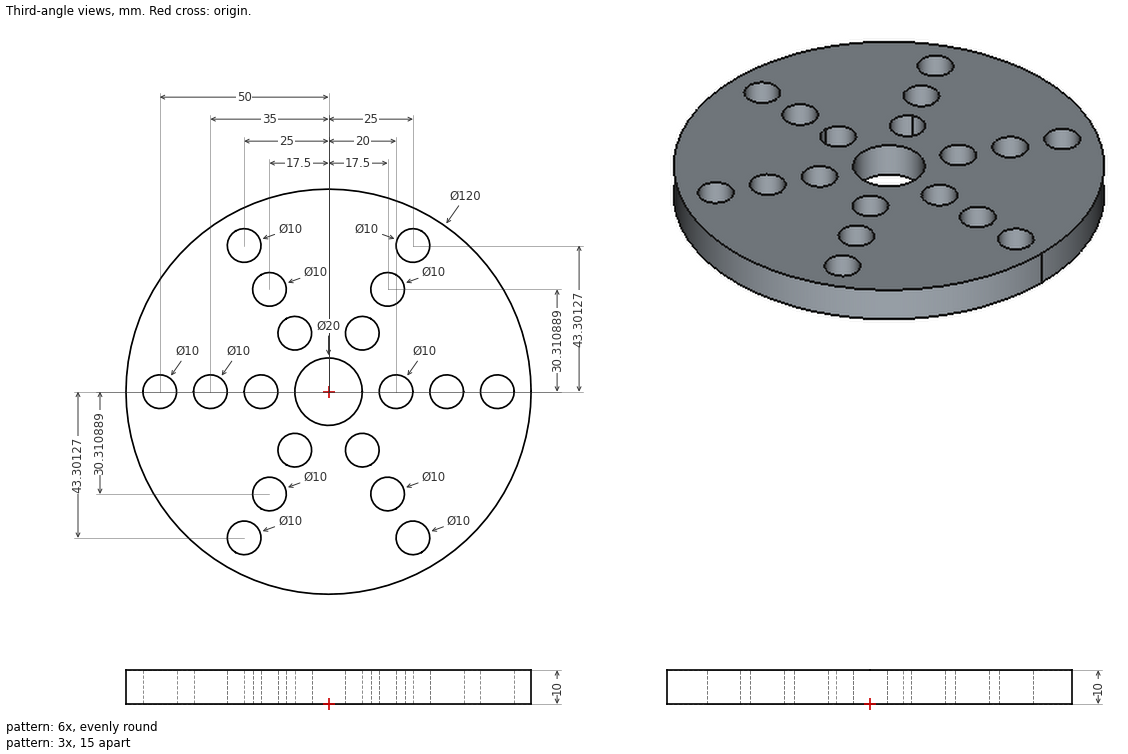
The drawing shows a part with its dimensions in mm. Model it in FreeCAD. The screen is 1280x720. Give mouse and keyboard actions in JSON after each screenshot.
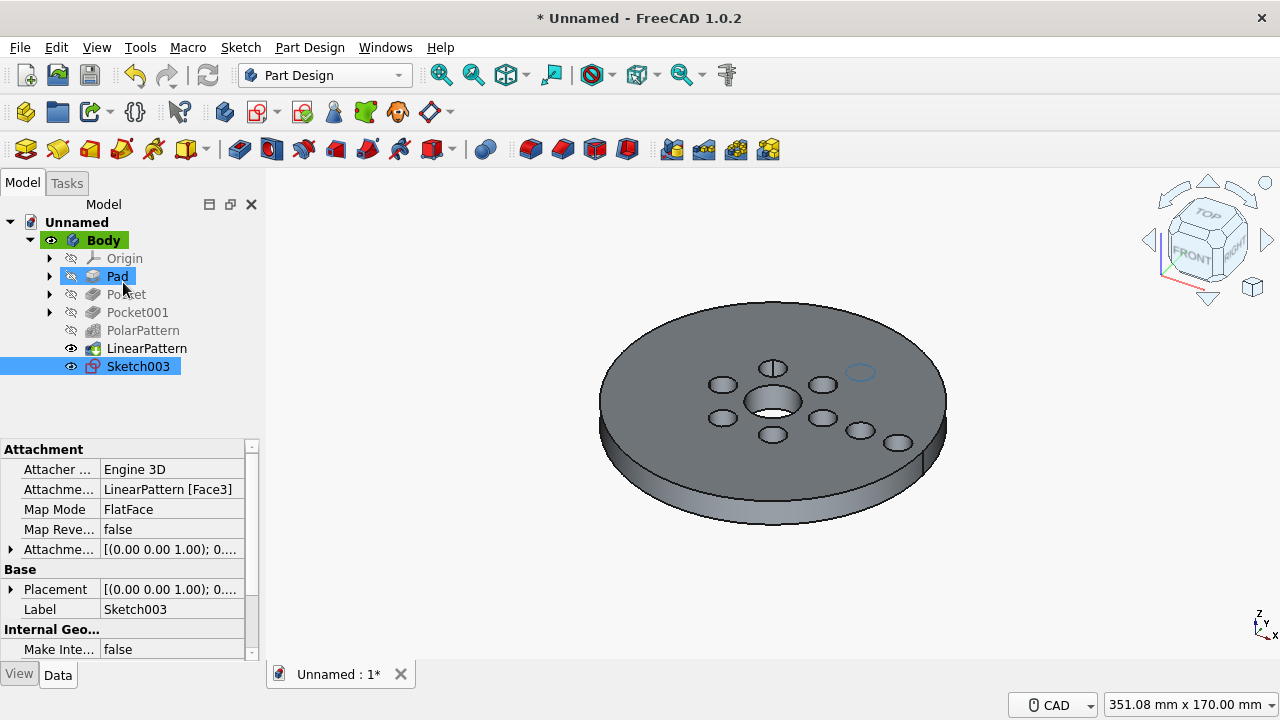
{"action": "left_click", "coordinate": [240, 150]}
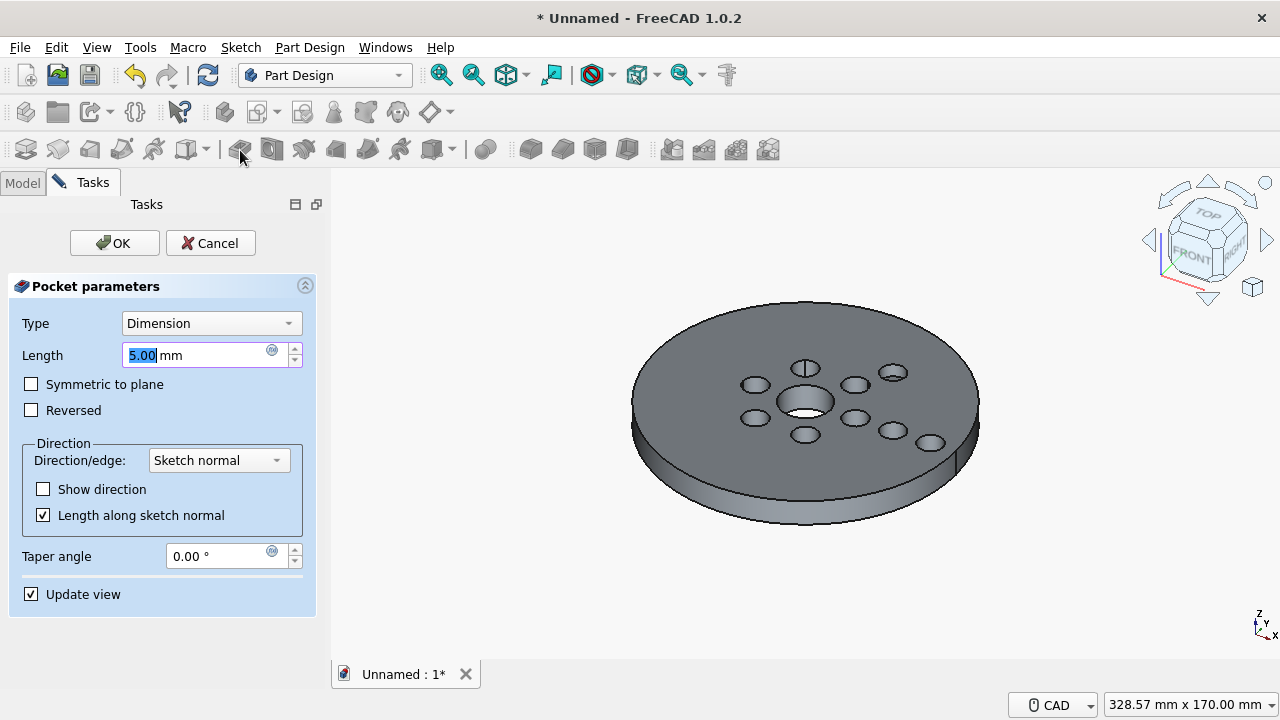
{"action": "type", "text": "10"}
{"action": "key", "text": "Tab"}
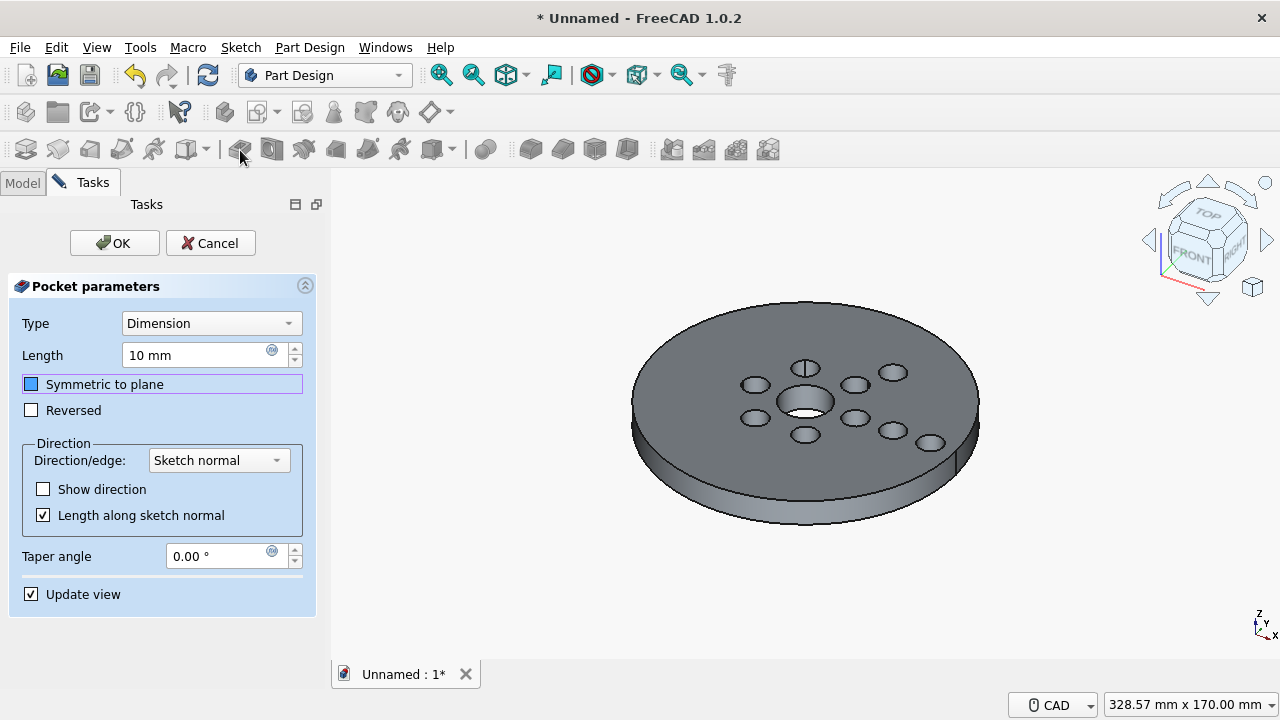
{"action": "left_click", "coordinate": [115, 243]}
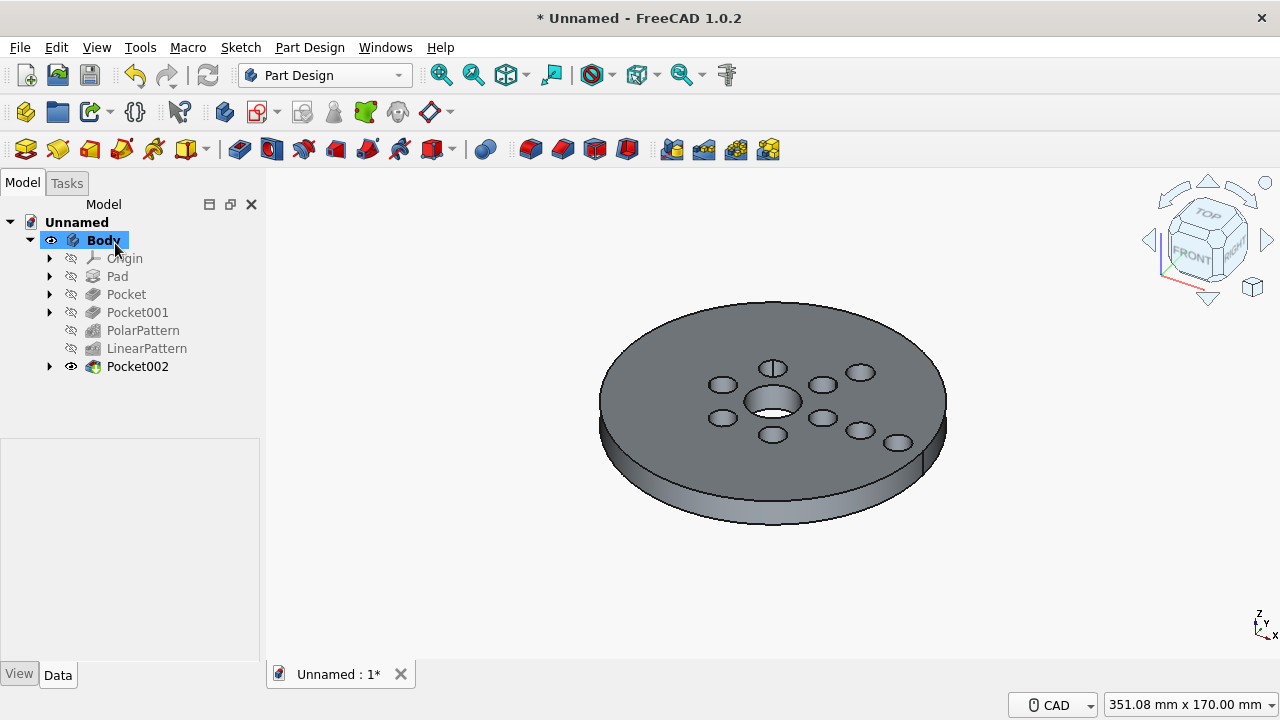
{"action": "left_click", "coordinate": [662, 397]}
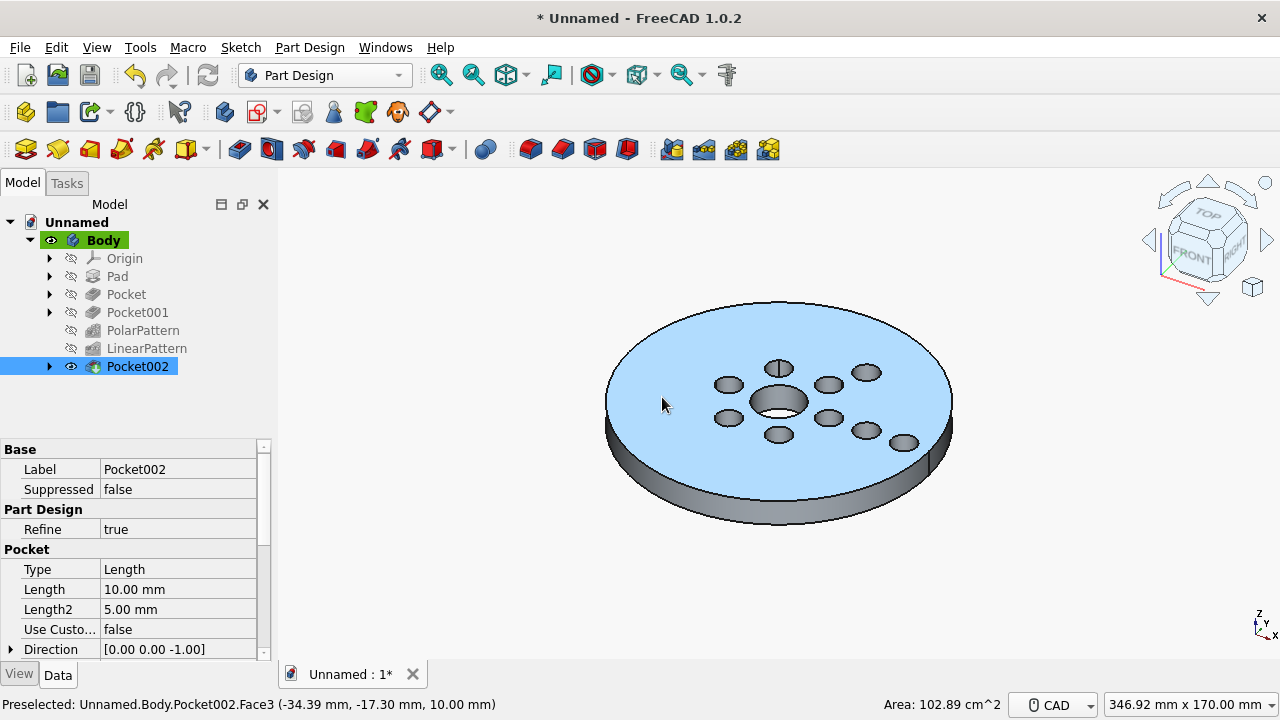
{"action": "left_click", "coordinate": [258, 112]}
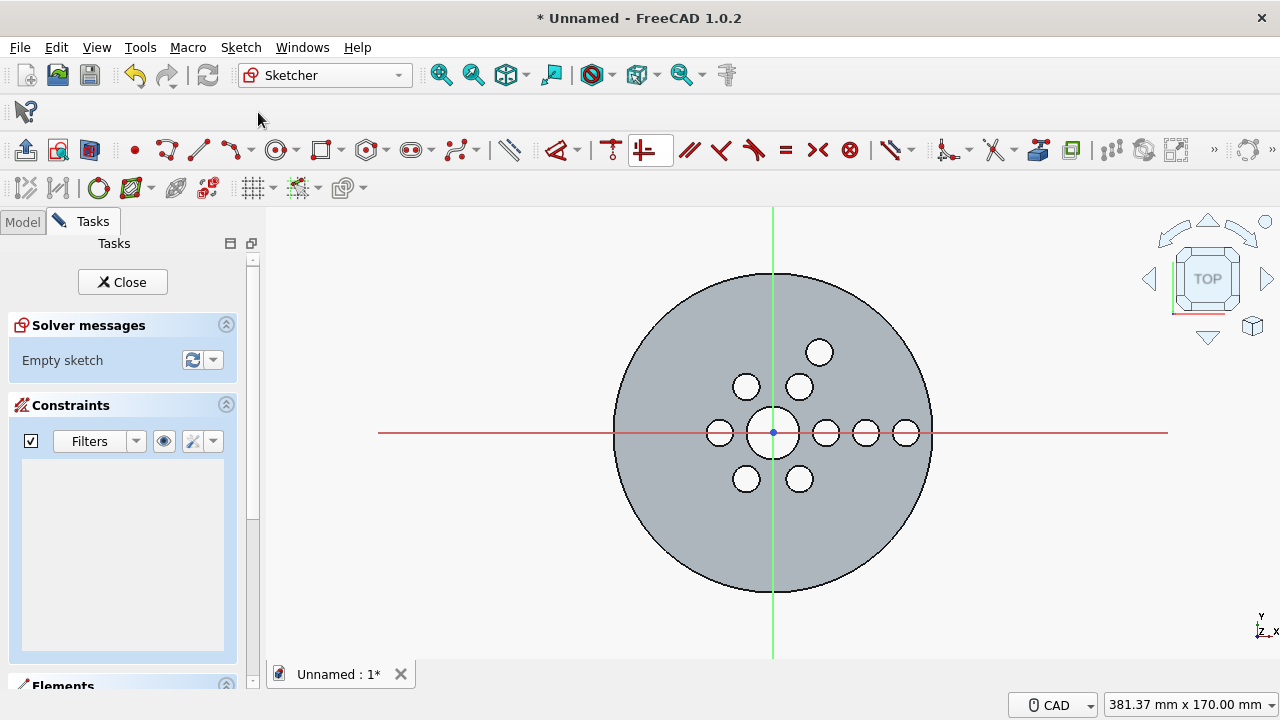
{"action": "scroll", "coordinate": [729, 344], "scroll_direction": "up", "scroll_amount": 12}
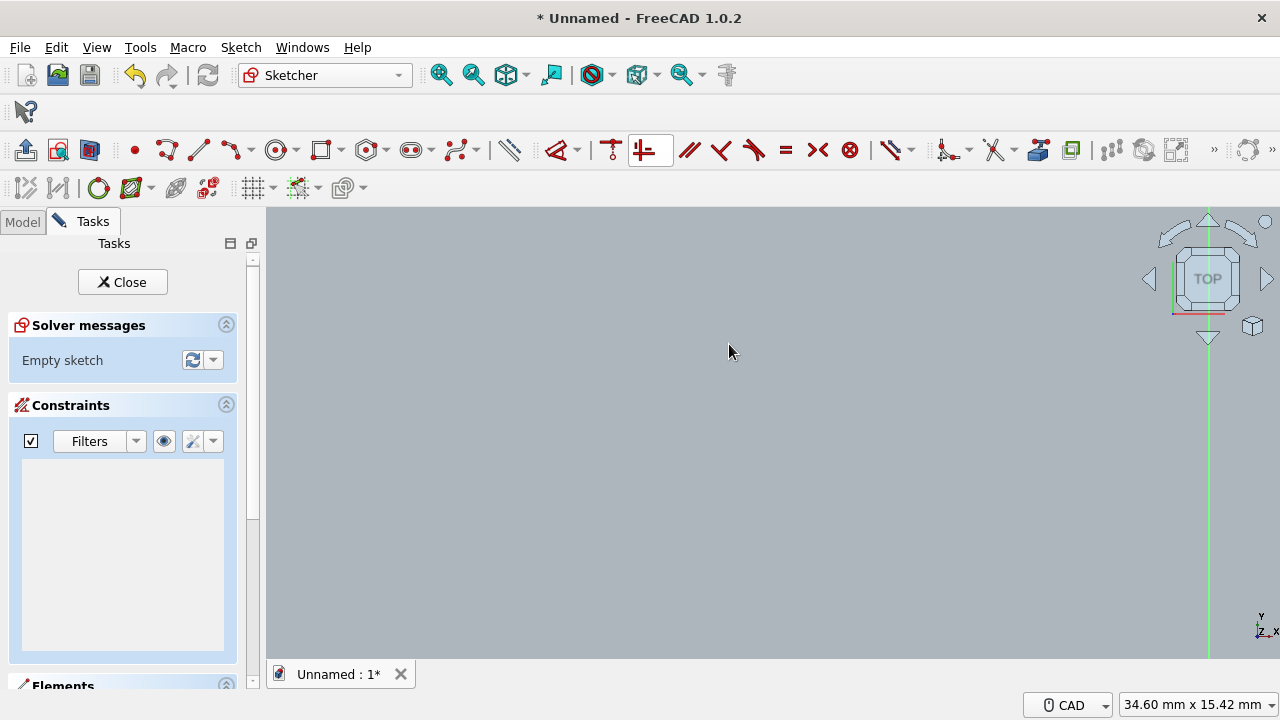
{"action": "left_click", "coordinate": [276, 150]}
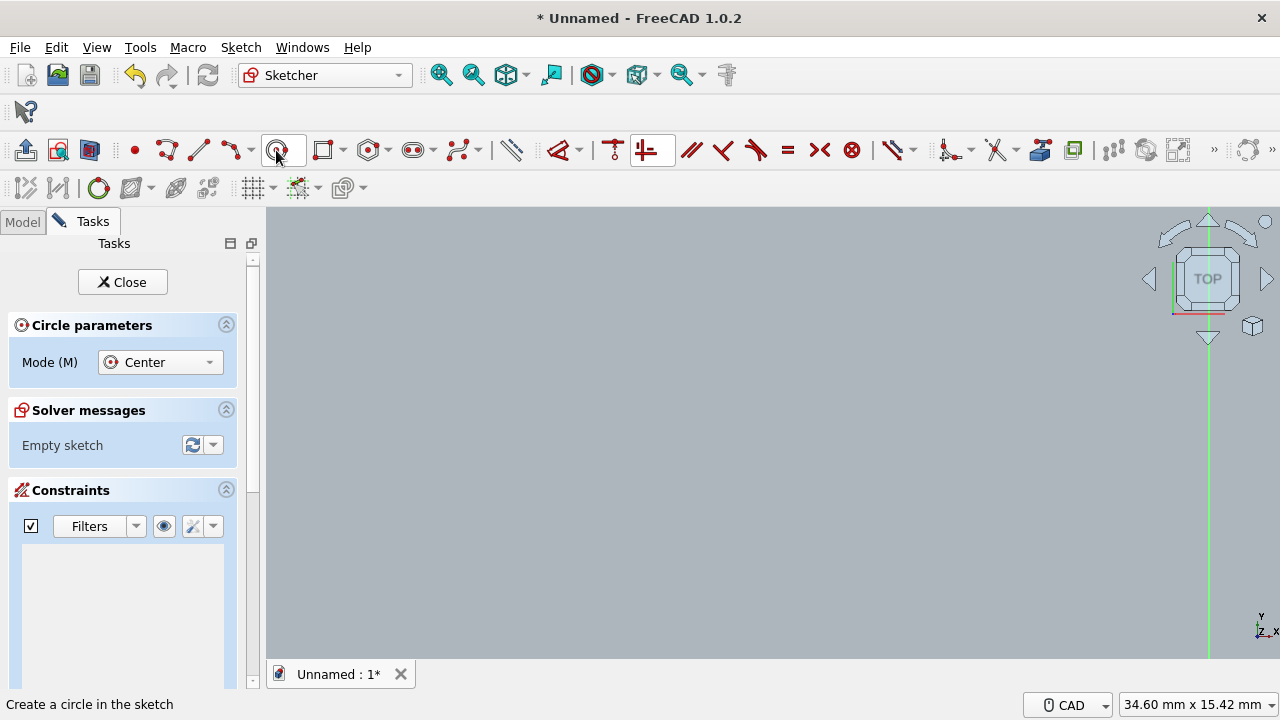
{"action": "left_click", "coordinate": [697, 434]}
{"action": "left_click", "coordinate": [800, 330]}
{"action": "key", "text": "Escape"}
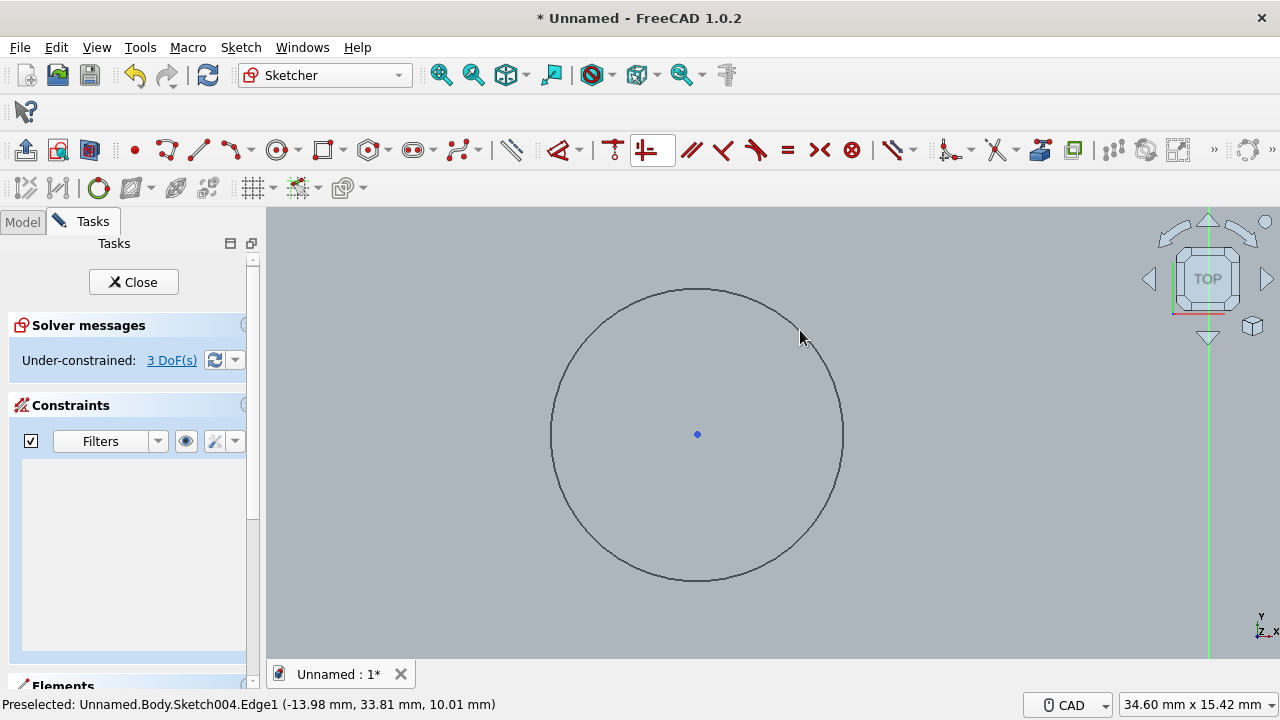
{"action": "left_click", "coordinate": [558, 150]}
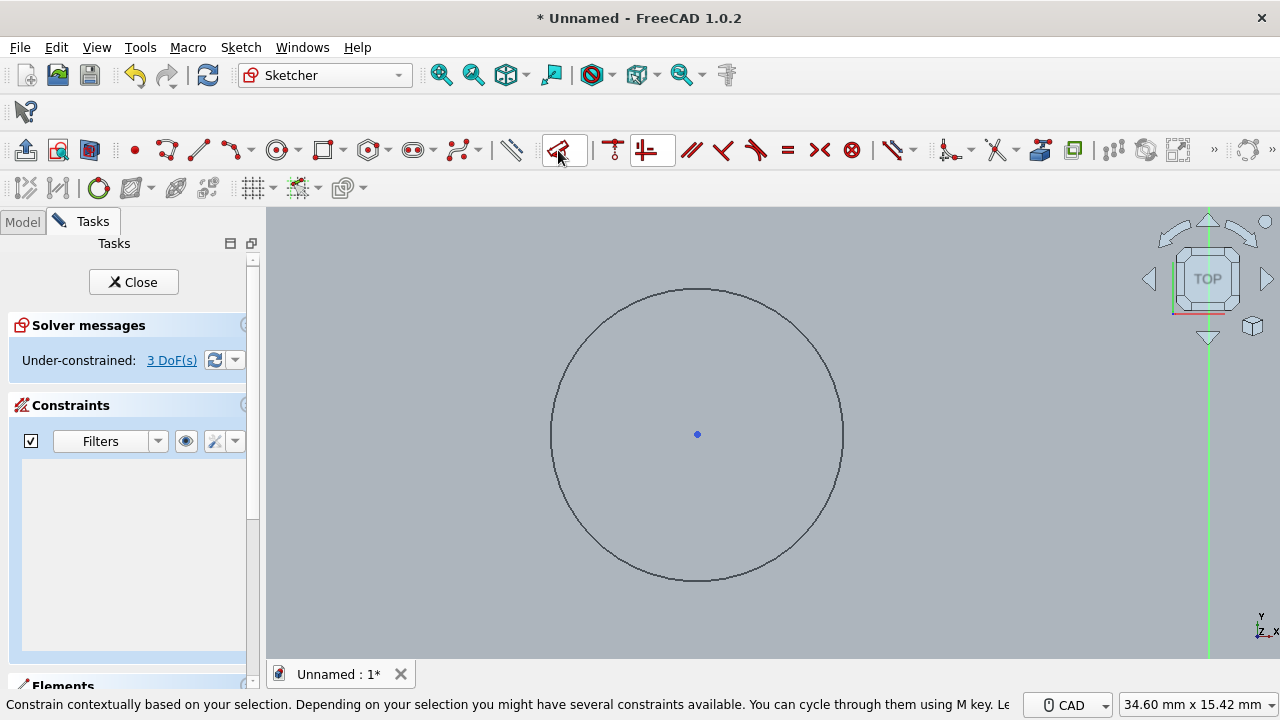
{"action": "left_click", "coordinate": [800, 331]}
{"action": "left_click", "coordinate": [823, 308]}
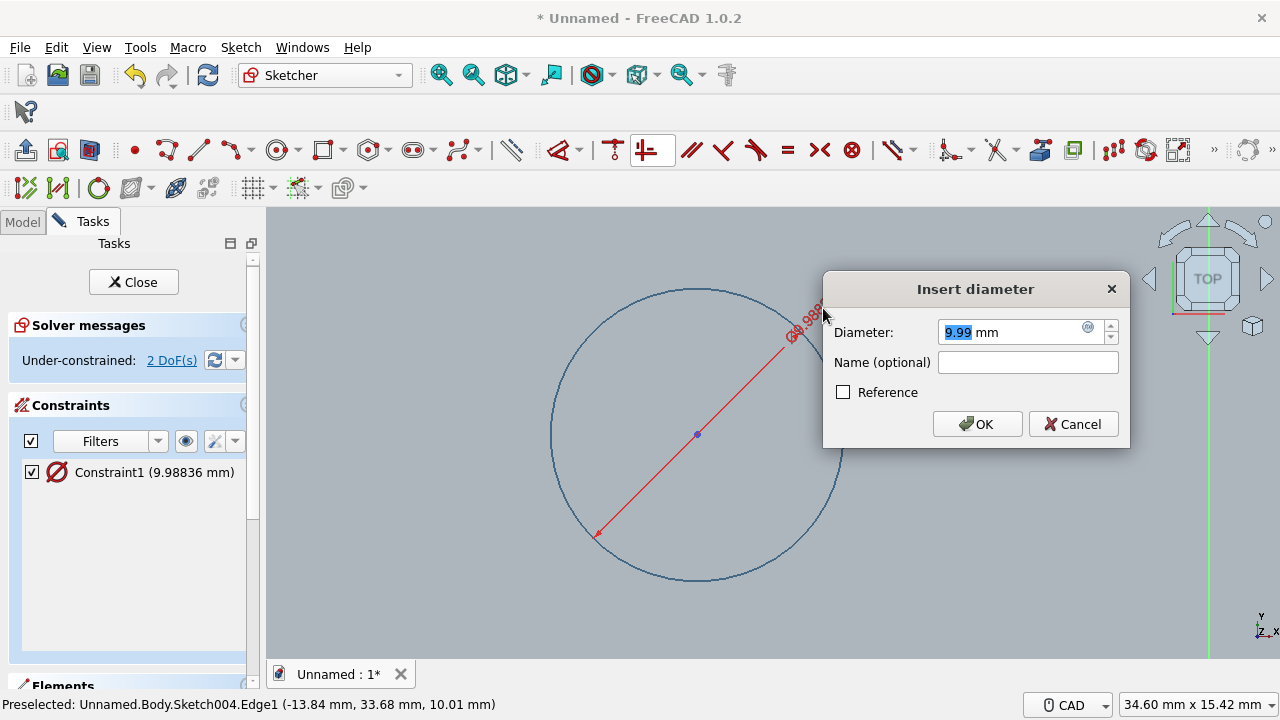
{"action": "type", "text": "10"}
{"action": "key", "text": "Return"}